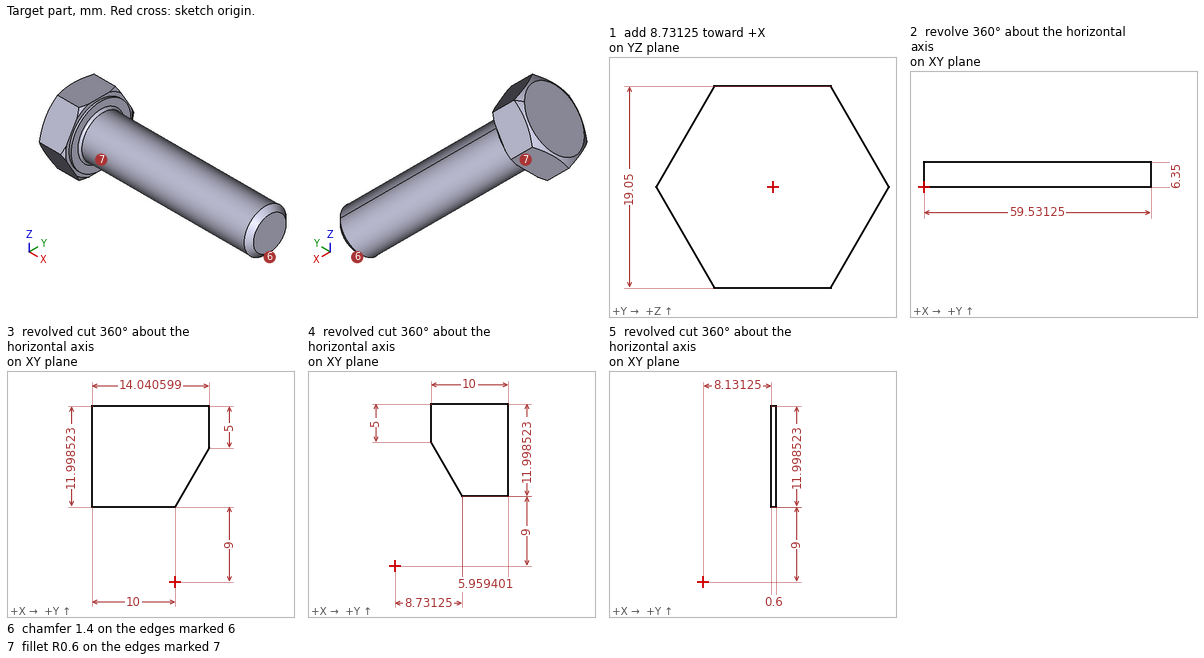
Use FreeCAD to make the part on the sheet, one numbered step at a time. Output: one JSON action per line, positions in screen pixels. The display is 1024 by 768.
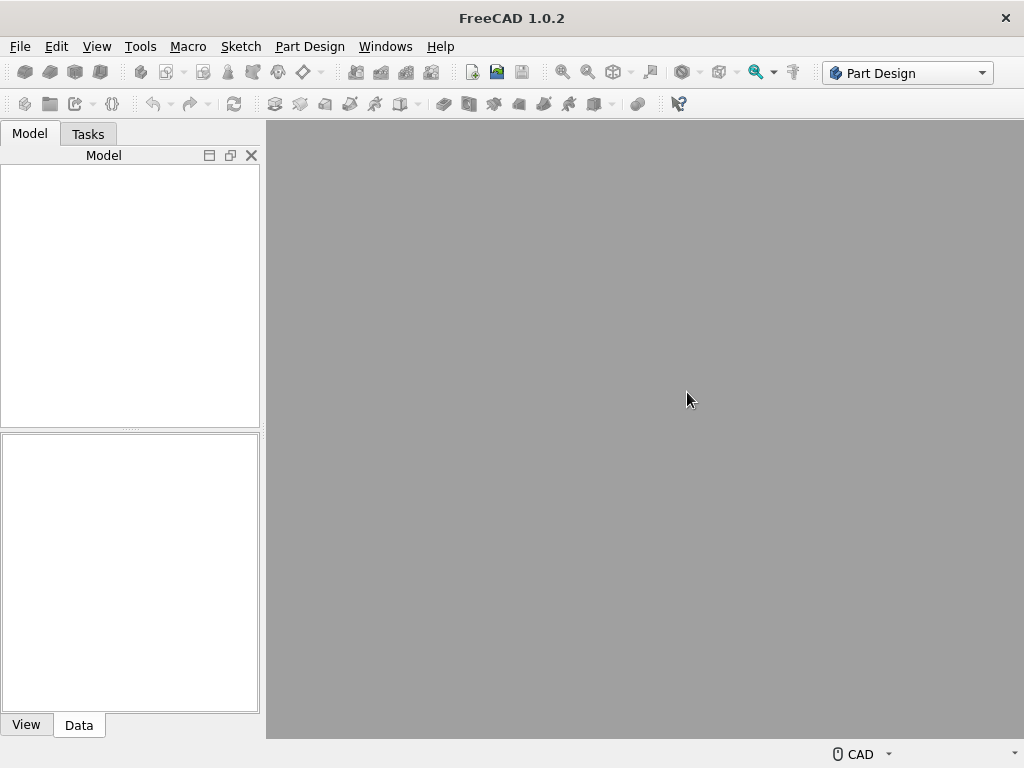
{"action": "left_click", "coordinate": [472, 72]}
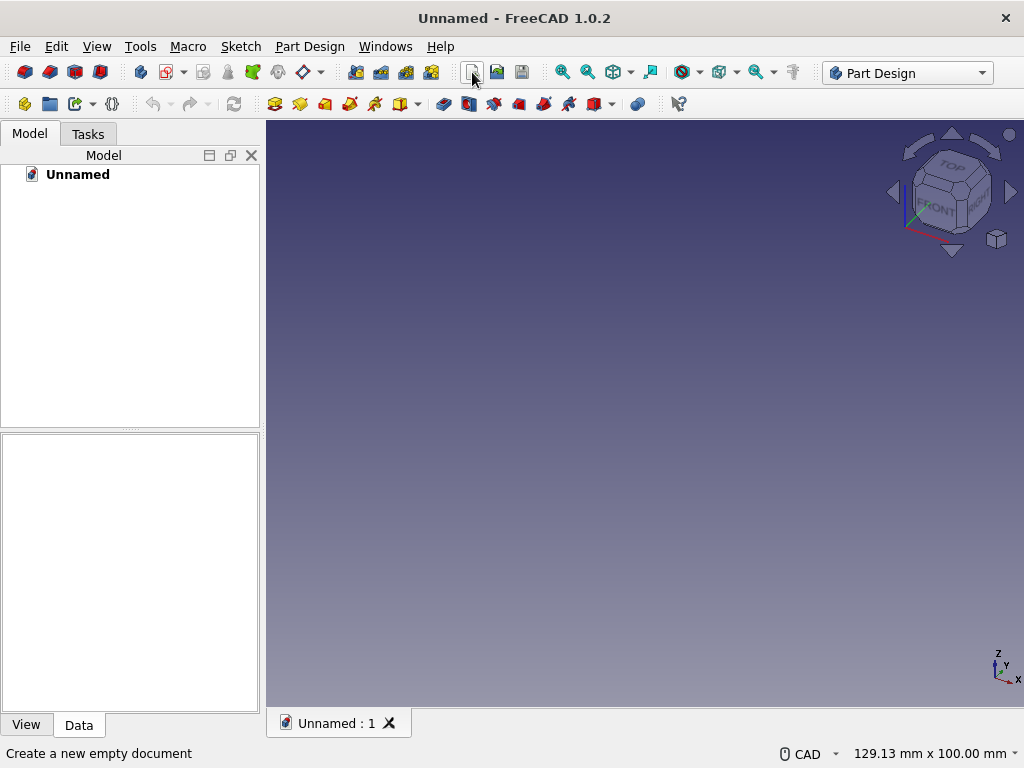
{"action": "left_click", "coordinate": [166, 72]}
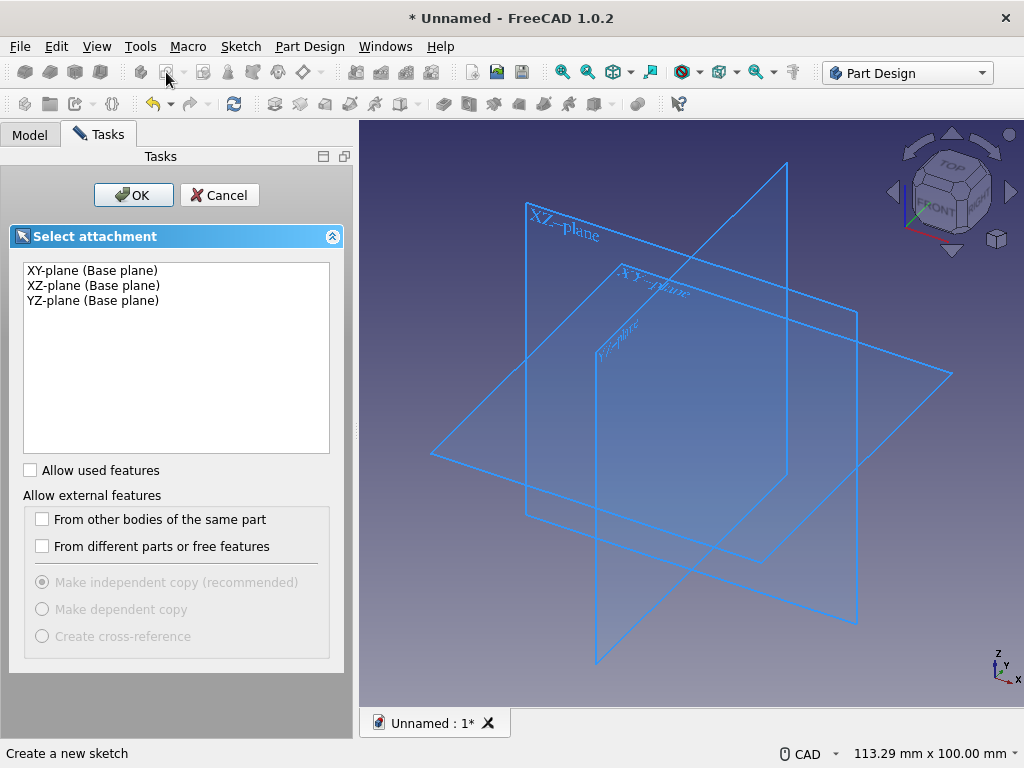
{"action": "left_click", "coordinate": [84, 300]}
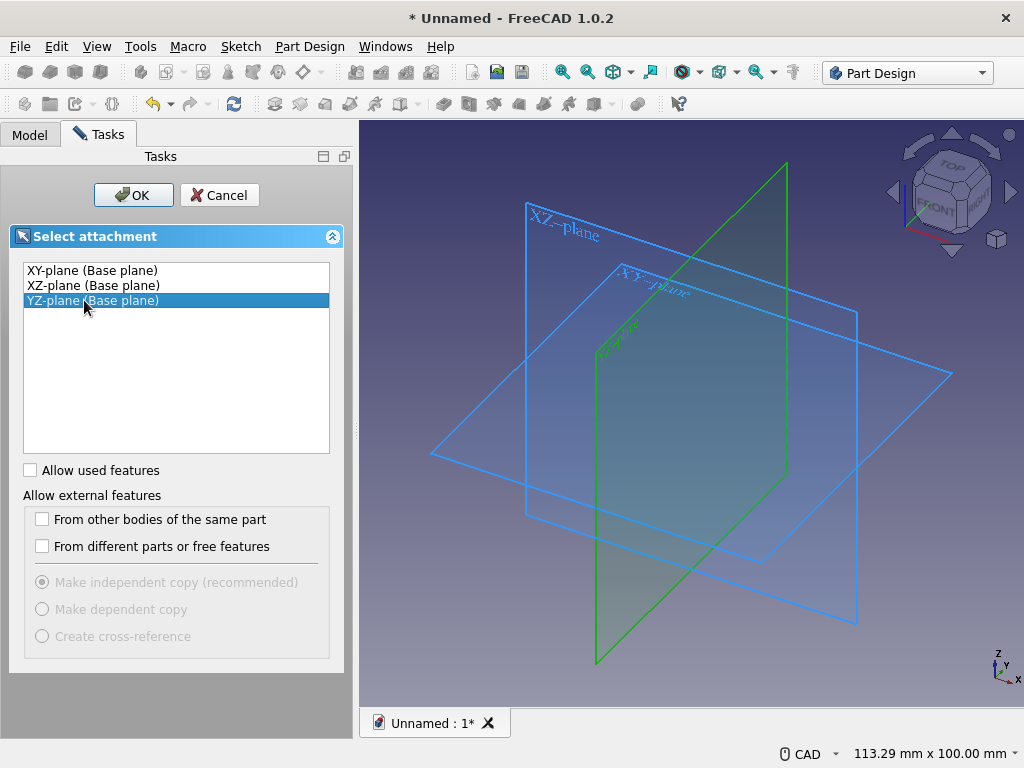
{"action": "left_click", "coordinate": [134, 195]}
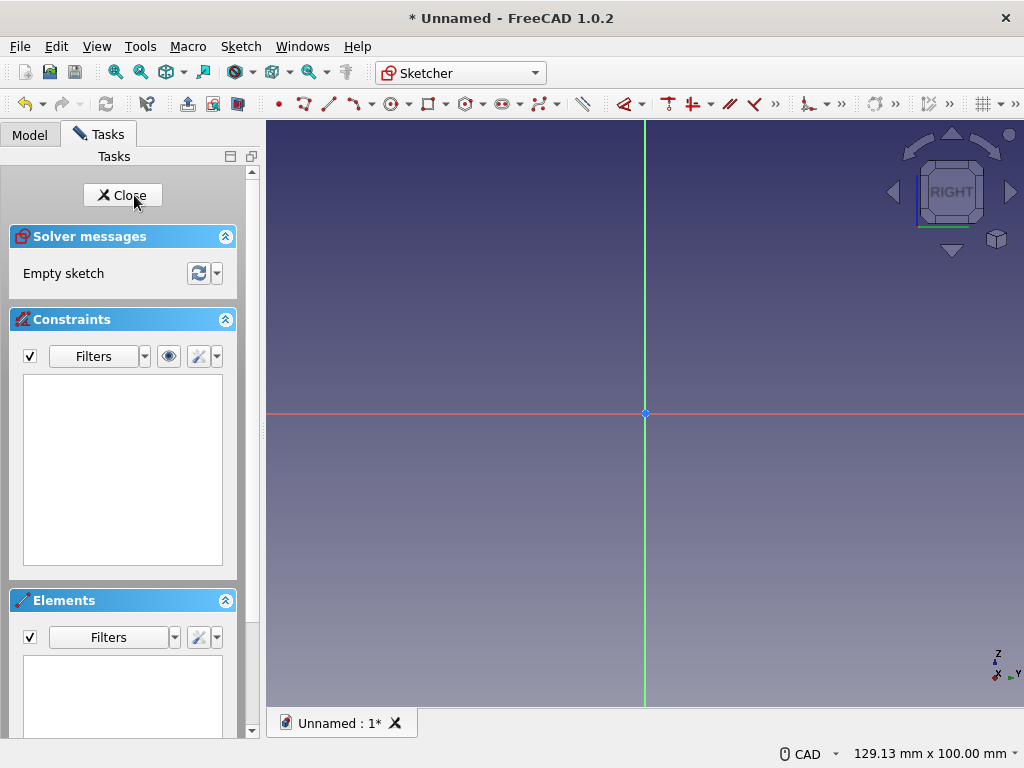
{"action": "scroll", "coordinate": [675, 414], "scroll_direction": "up", "scroll_amount": 6}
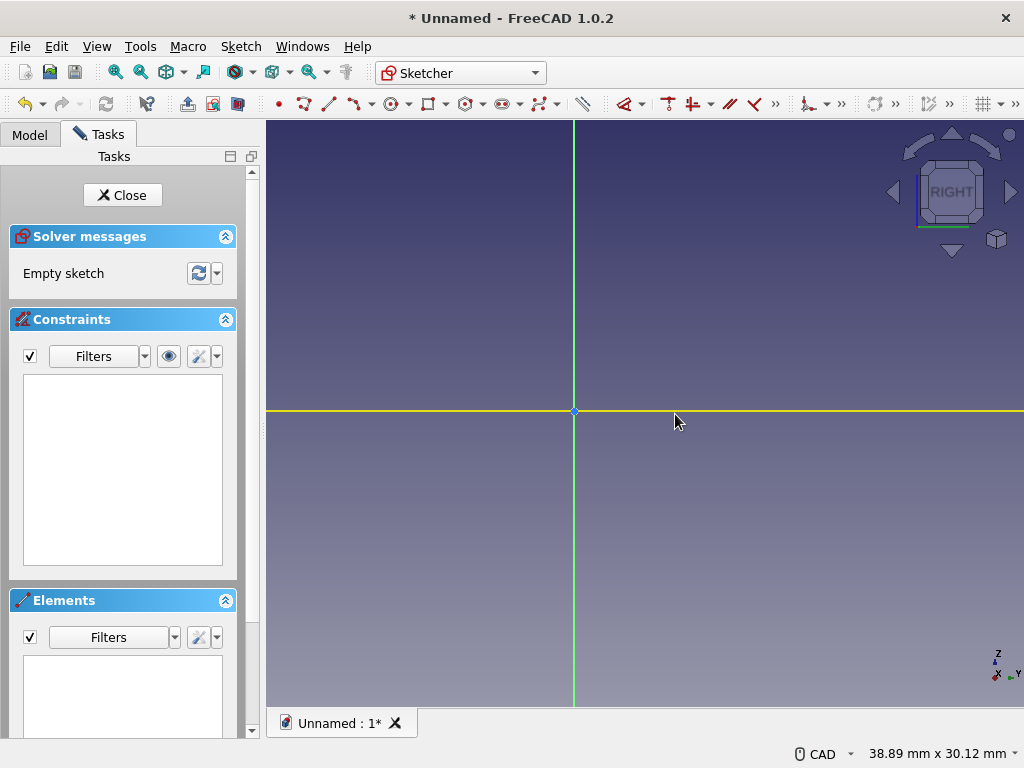
{"action": "left_click", "coordinate": [464, 104]}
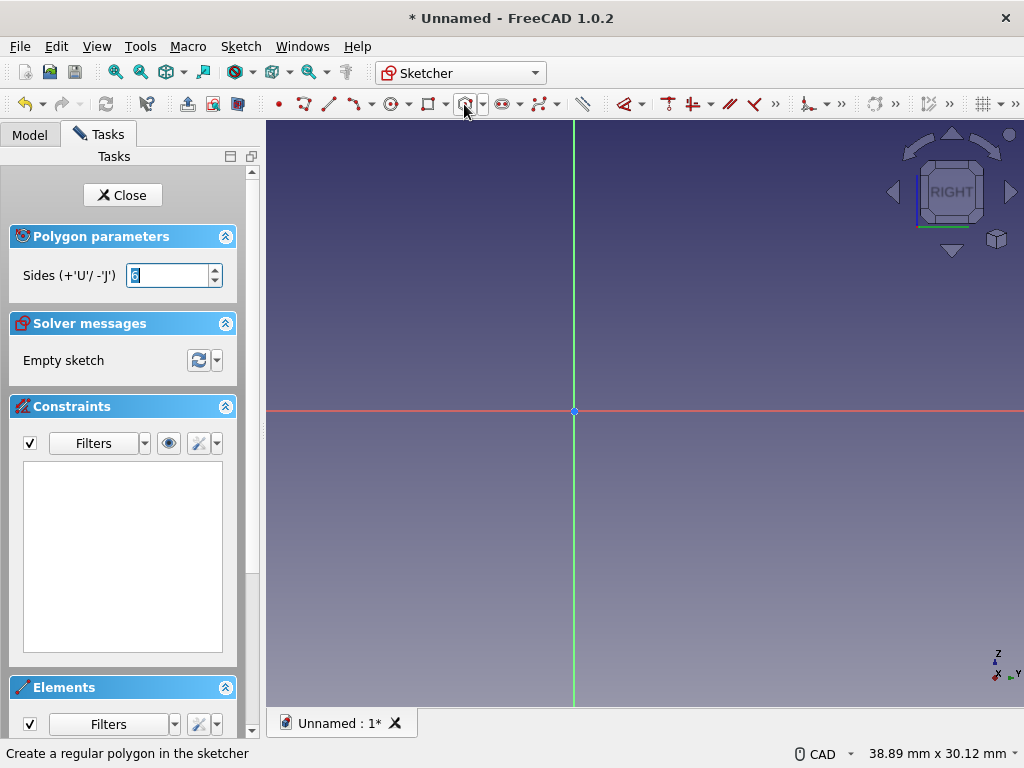
{"action": "left_click", "coordinate": [574, 411]}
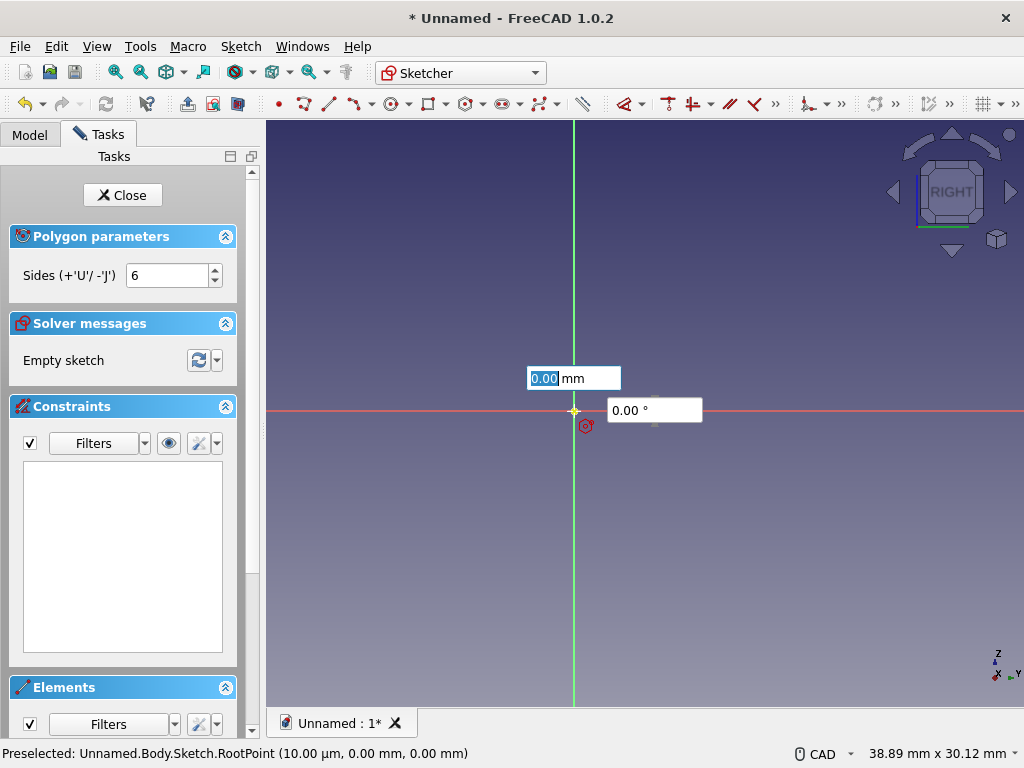
{"action": "left_click", "coordinate": [788, 411]}
{"action": "right_click", "coordinate": [788, 411]}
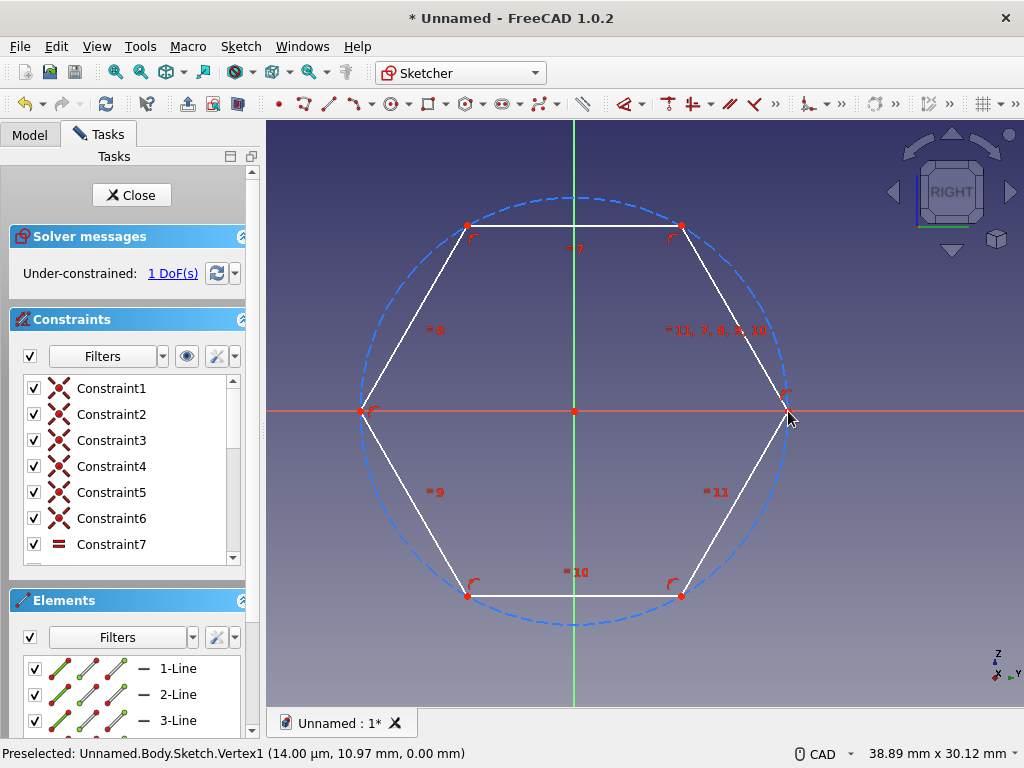
{"action": "left_click", "coordinate": [624, 104]}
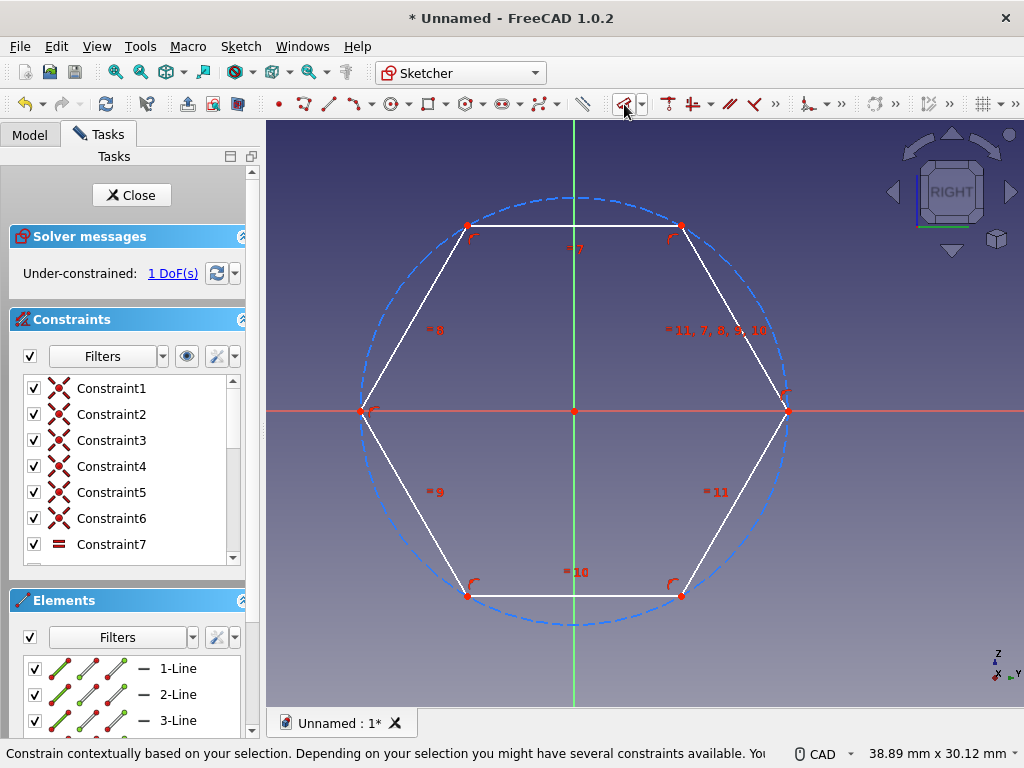
{"action": "left_click", "coordinate": [467, 596]}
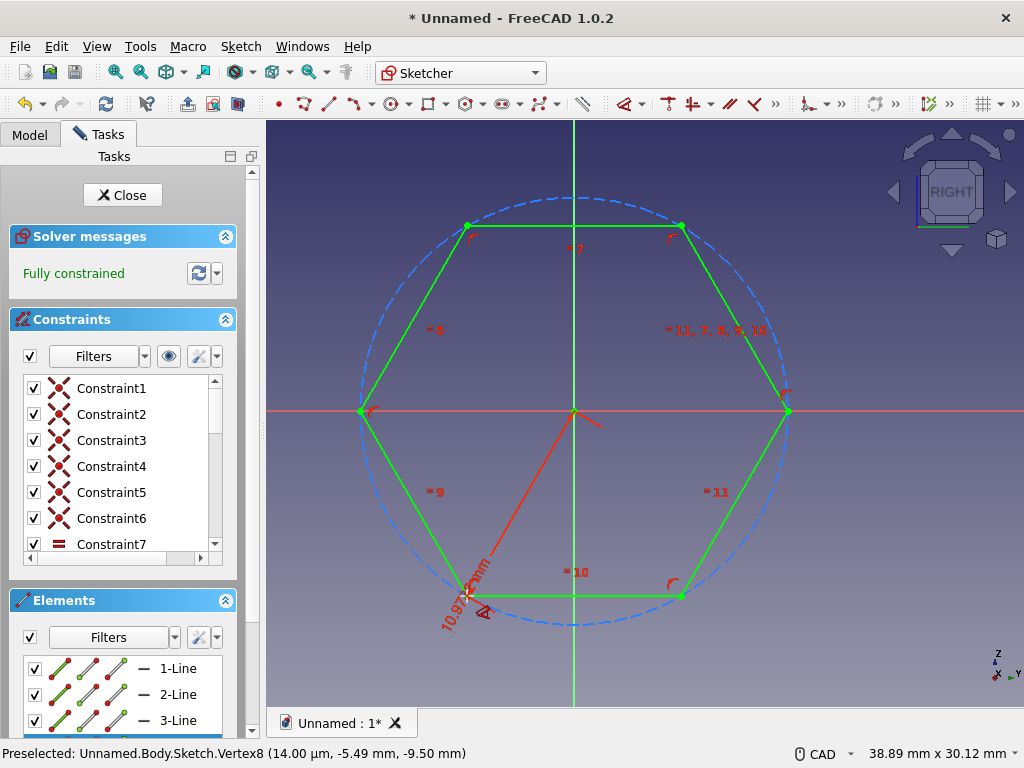
{"action": "left_click", "coordinate": [681, 226]}
{"action": "left_click", "coordinate": [715, 326]}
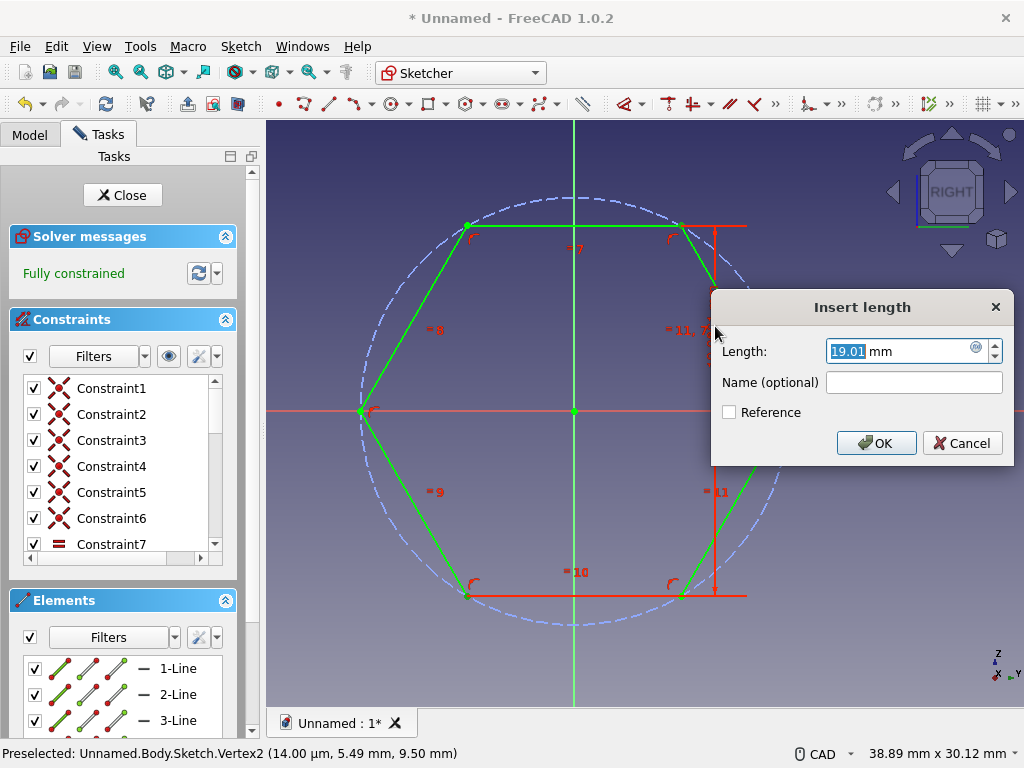
{"action": "type", "text": "19.05"}
{"action": "key", "text": "Return"}
{"action": "key", "text": "Escape"}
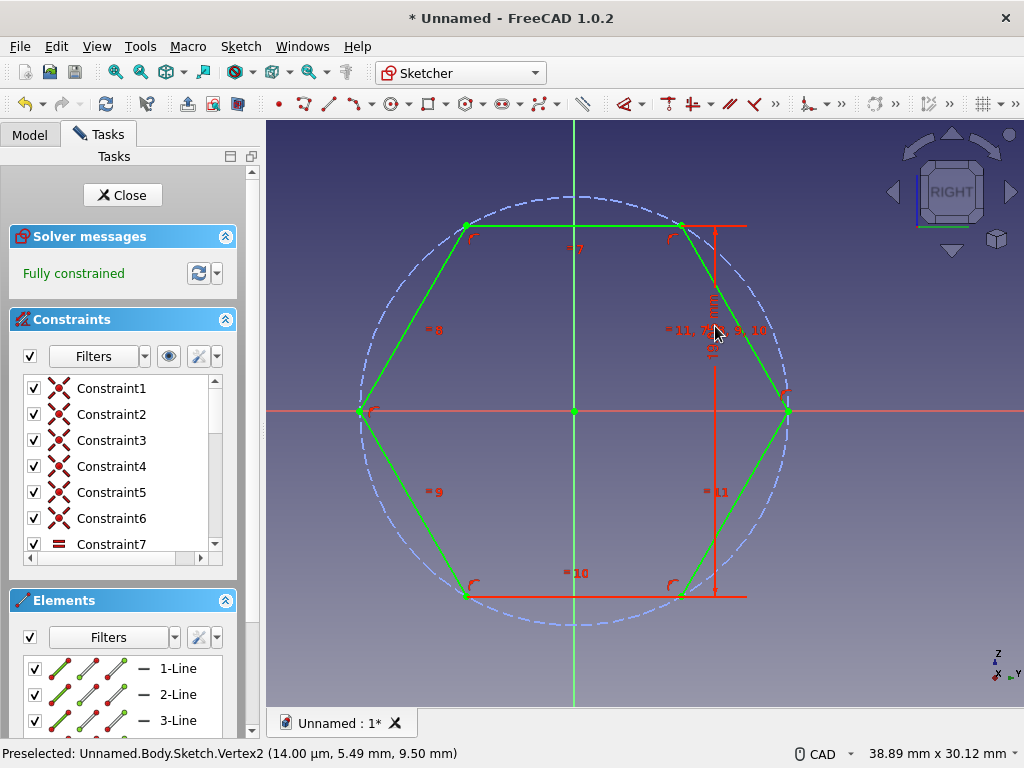
{"action": "left_click", "coordinate": [123, 195]}